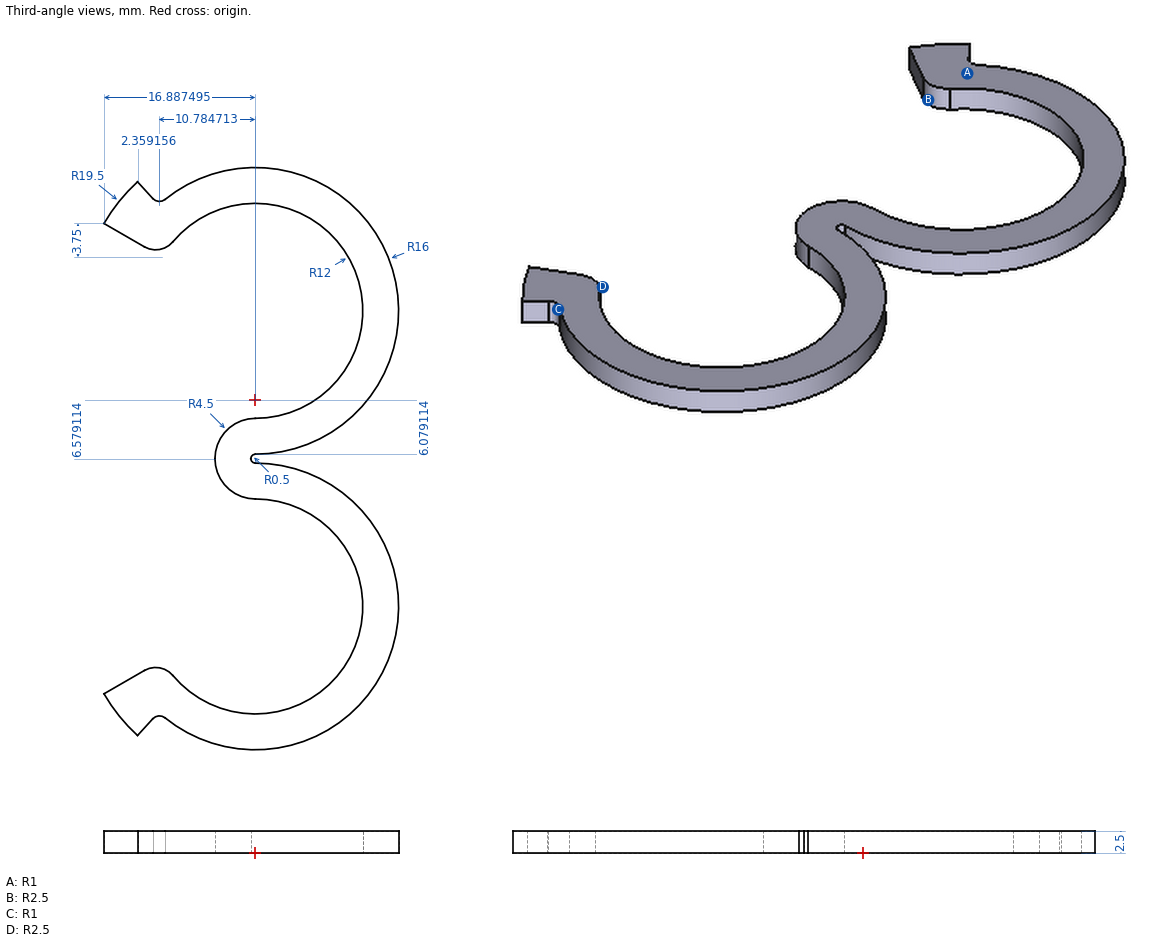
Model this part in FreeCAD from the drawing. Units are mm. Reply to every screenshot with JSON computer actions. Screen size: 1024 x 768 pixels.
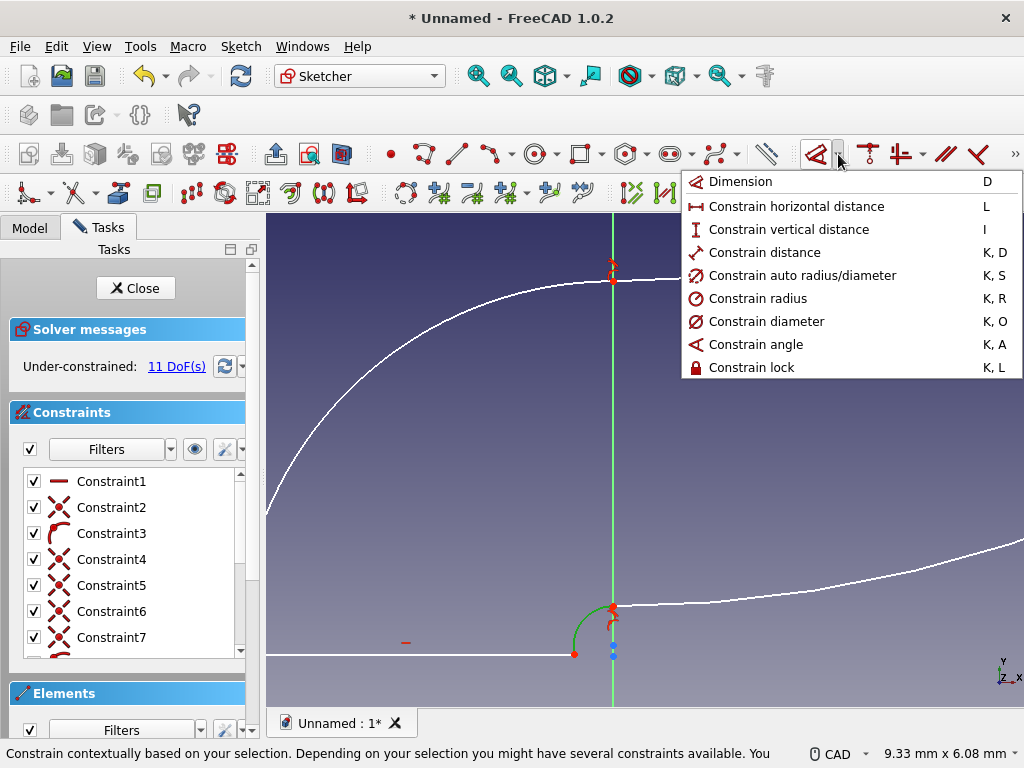
{"action": "left_click", "coordinate": [852, 298]}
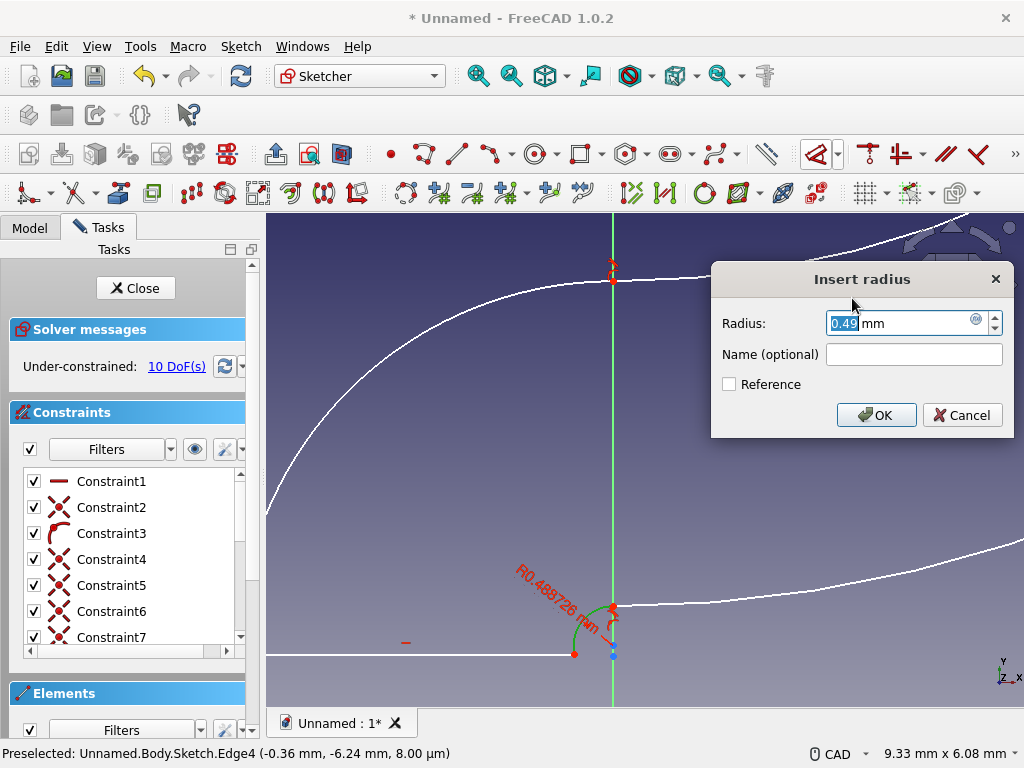
{"action": "type", "text": "0.5"}
{"action": "key", "text": "Return"}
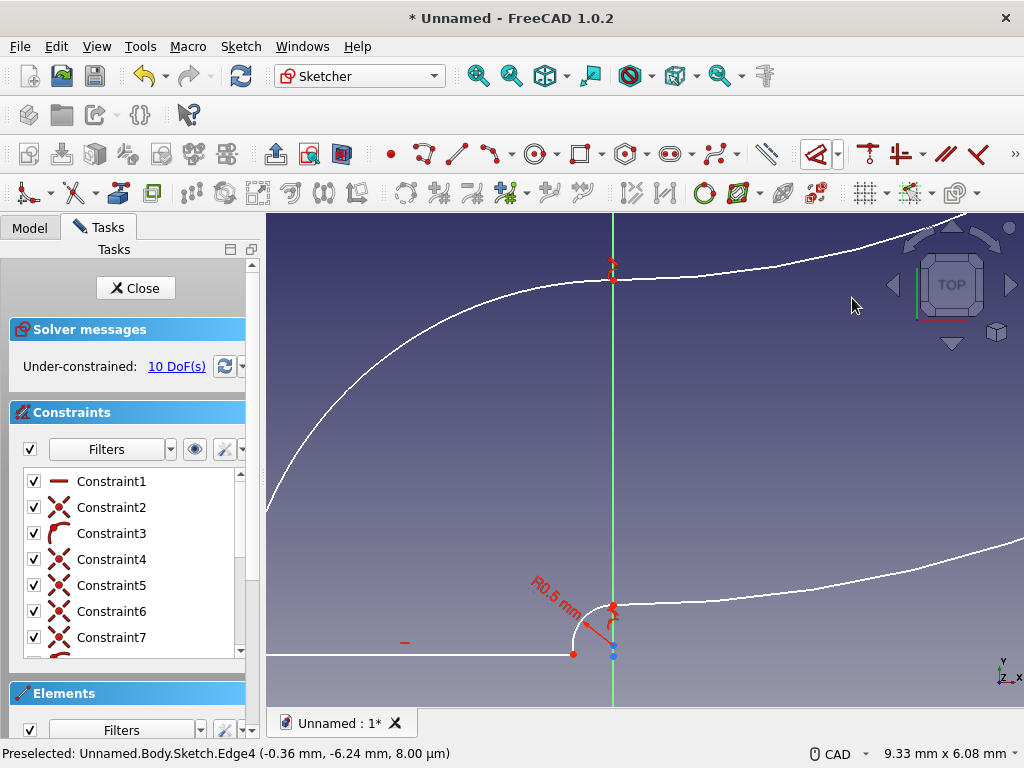
{"action": "scroll", "coordinate": [583, 627], "scroll_direction": "down", "scroll_amount": 10}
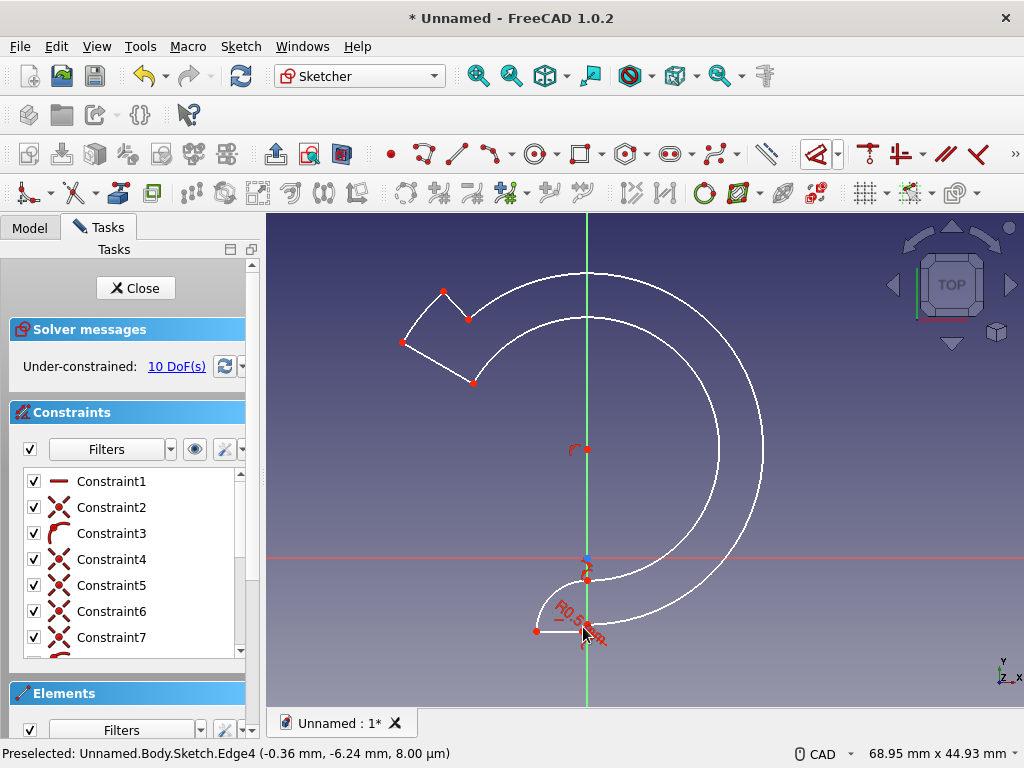
{"action": "left_click", "coordinate": [749, 518]}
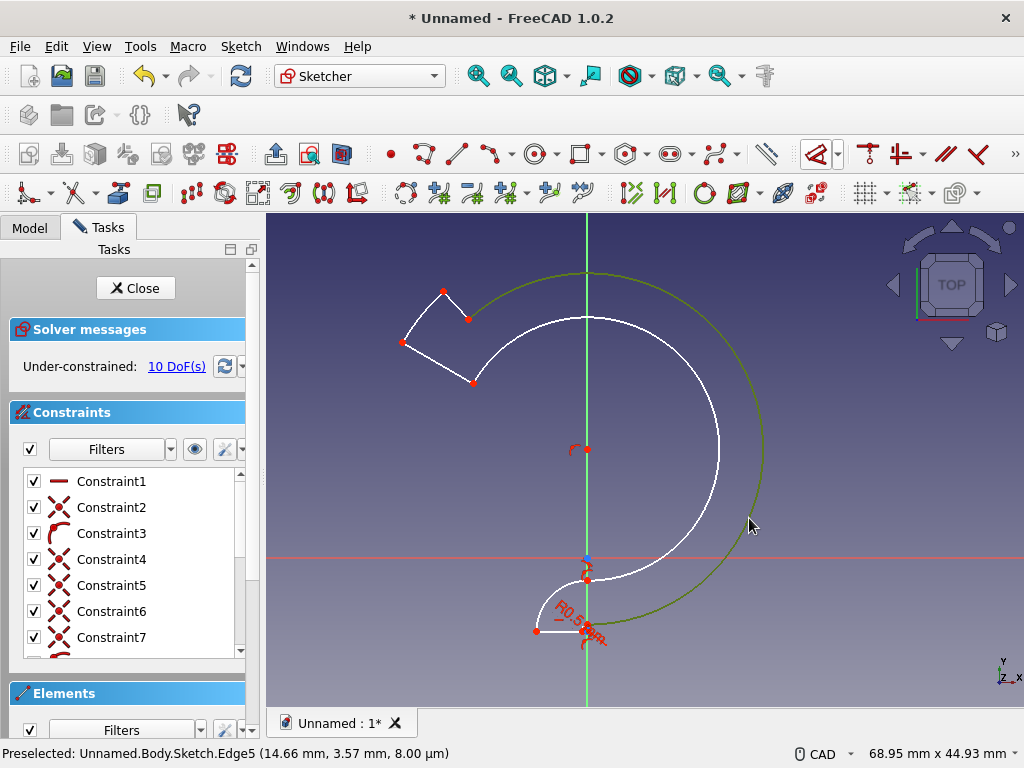
{"action": "key", "text": "k r"}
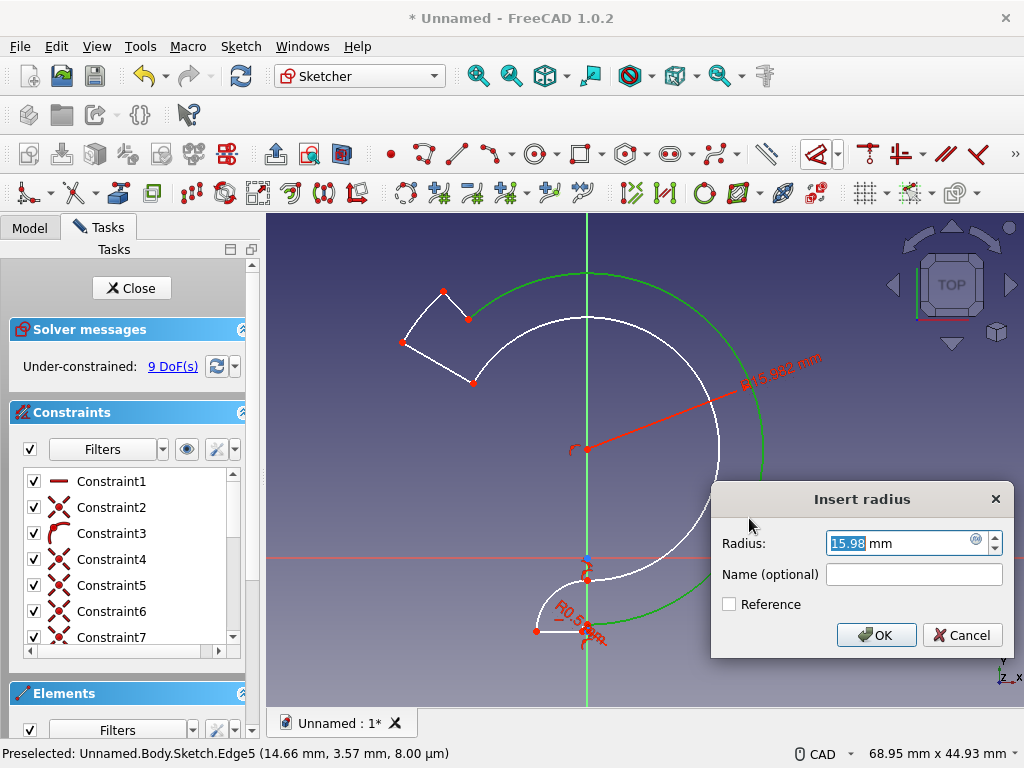
{"action": "type", "text": "16"}
{"action": "key", "text": "Return"}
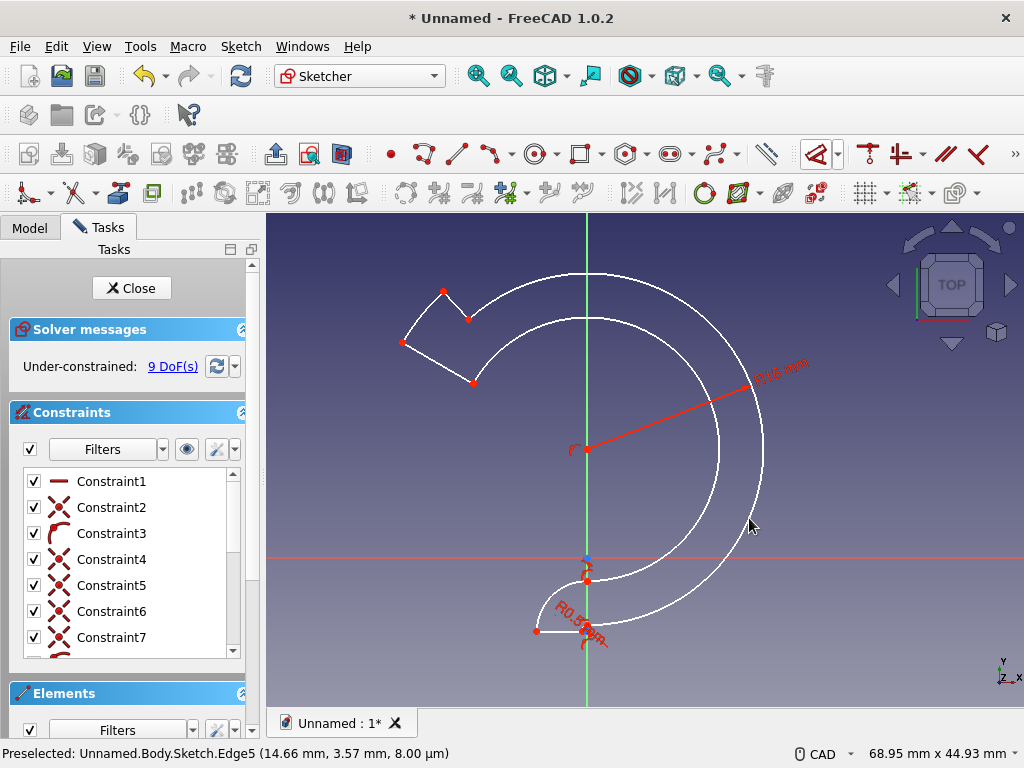
{"action": "left_click", "coordinate": [430, 306]}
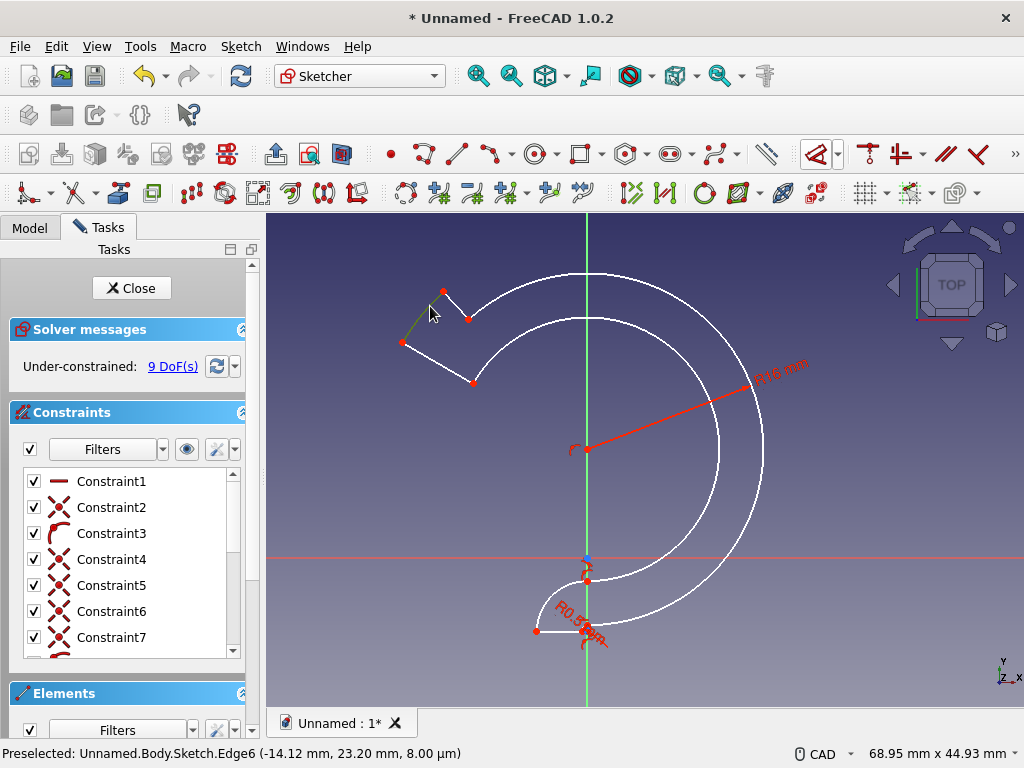
{"action": "key", "text": "k r"}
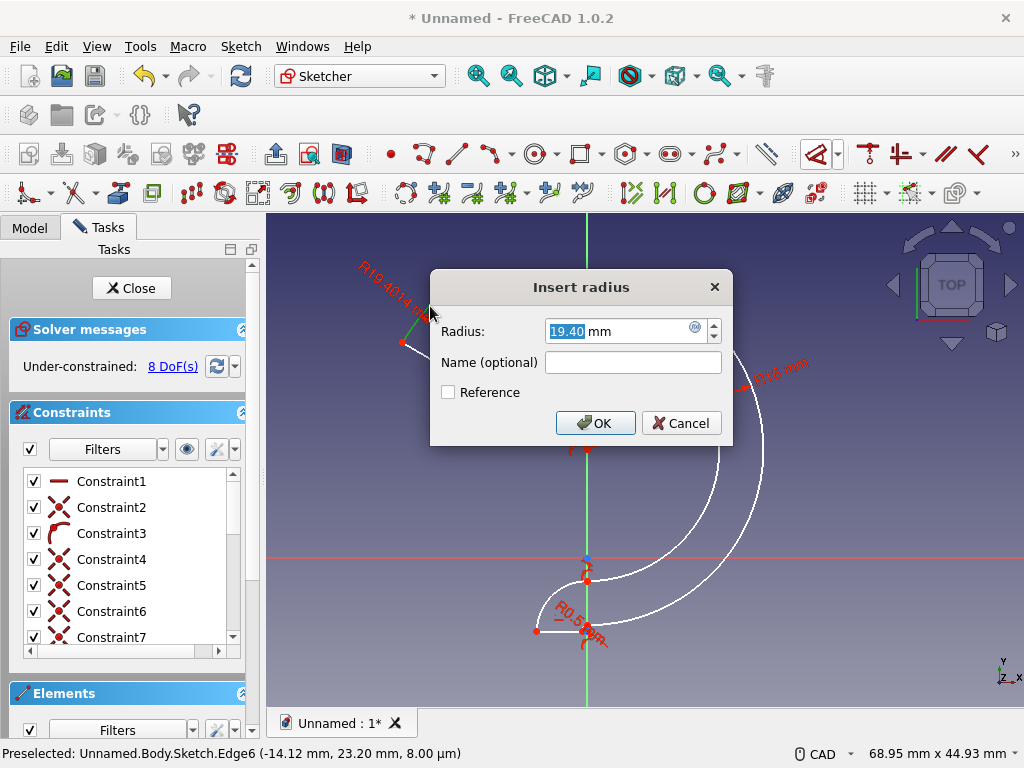
{"action": "type", "text": "19.5"}
{"action": "key", "text": "Return"}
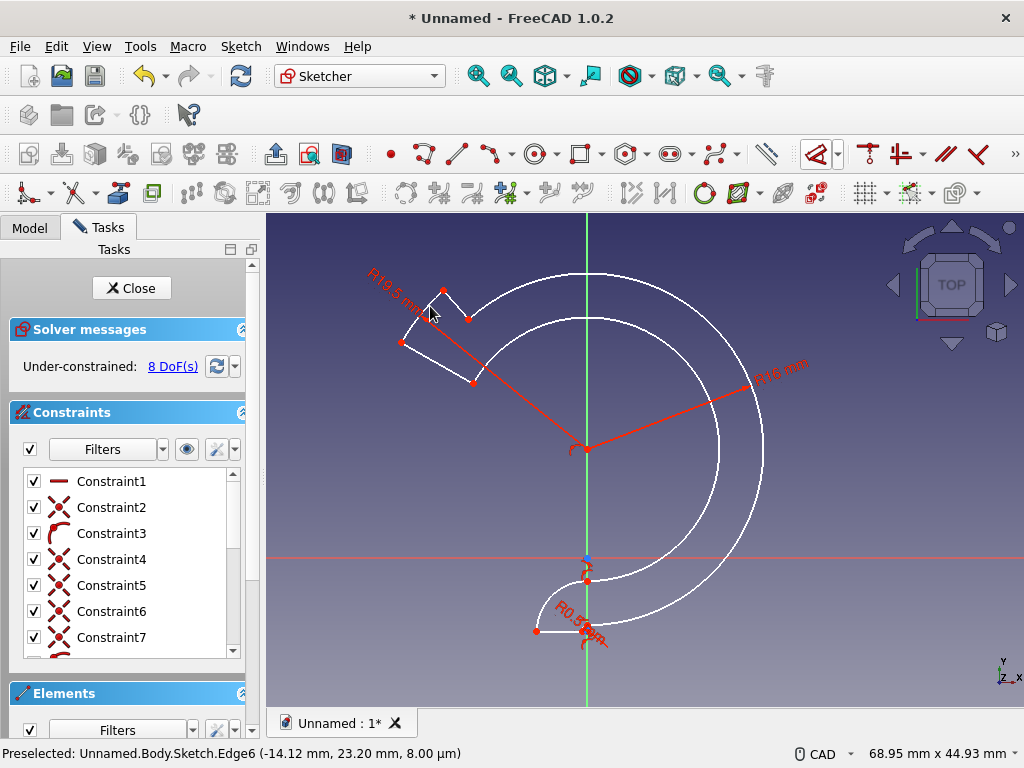
{"action": "left_click", "coordinate": [713, 490]}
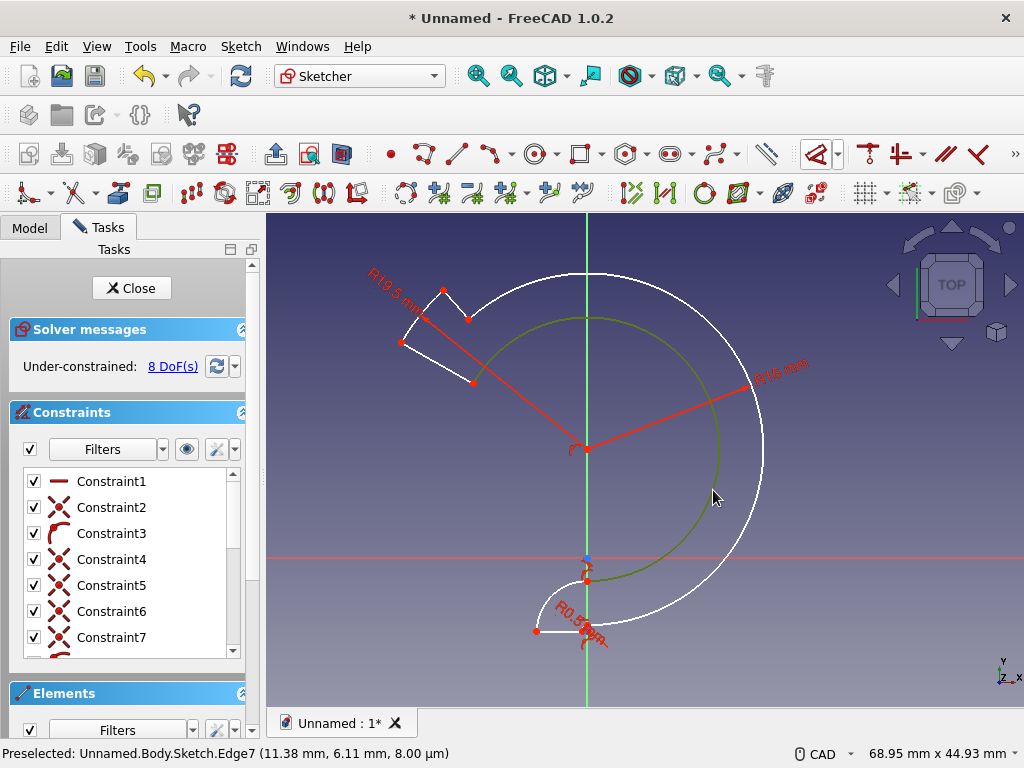
{"action": "key", "text": "k r"}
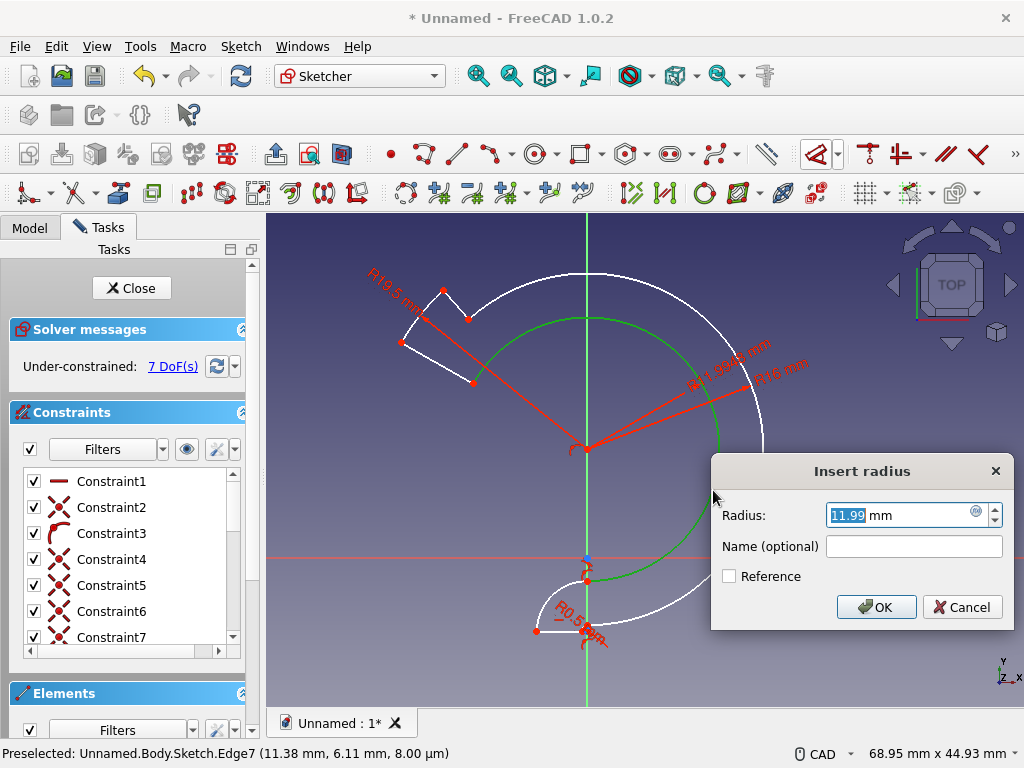
{"action": "type", "text": "12"}
{"action": "key", "text": "Return"}